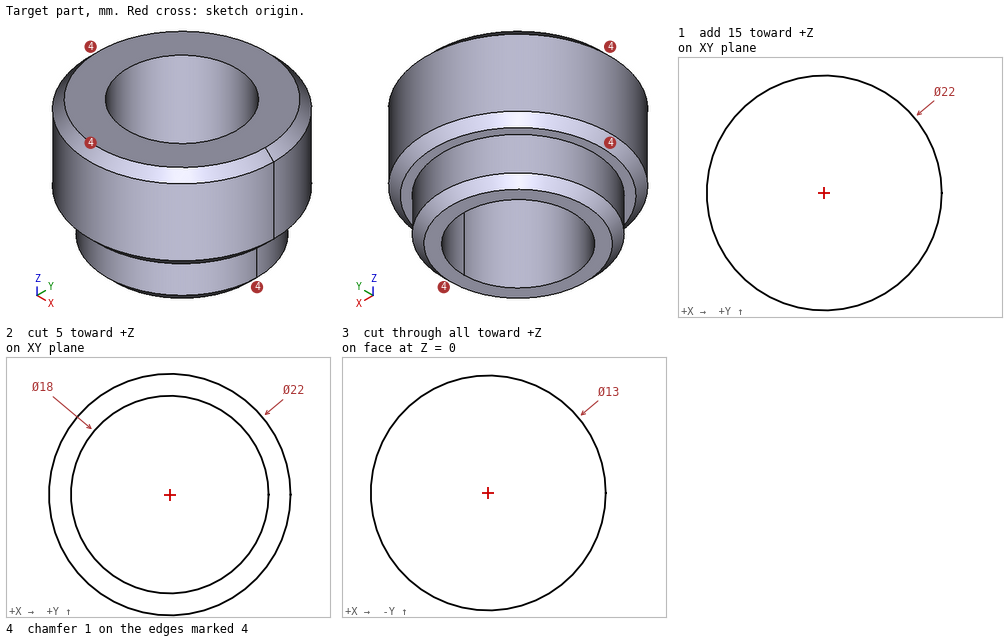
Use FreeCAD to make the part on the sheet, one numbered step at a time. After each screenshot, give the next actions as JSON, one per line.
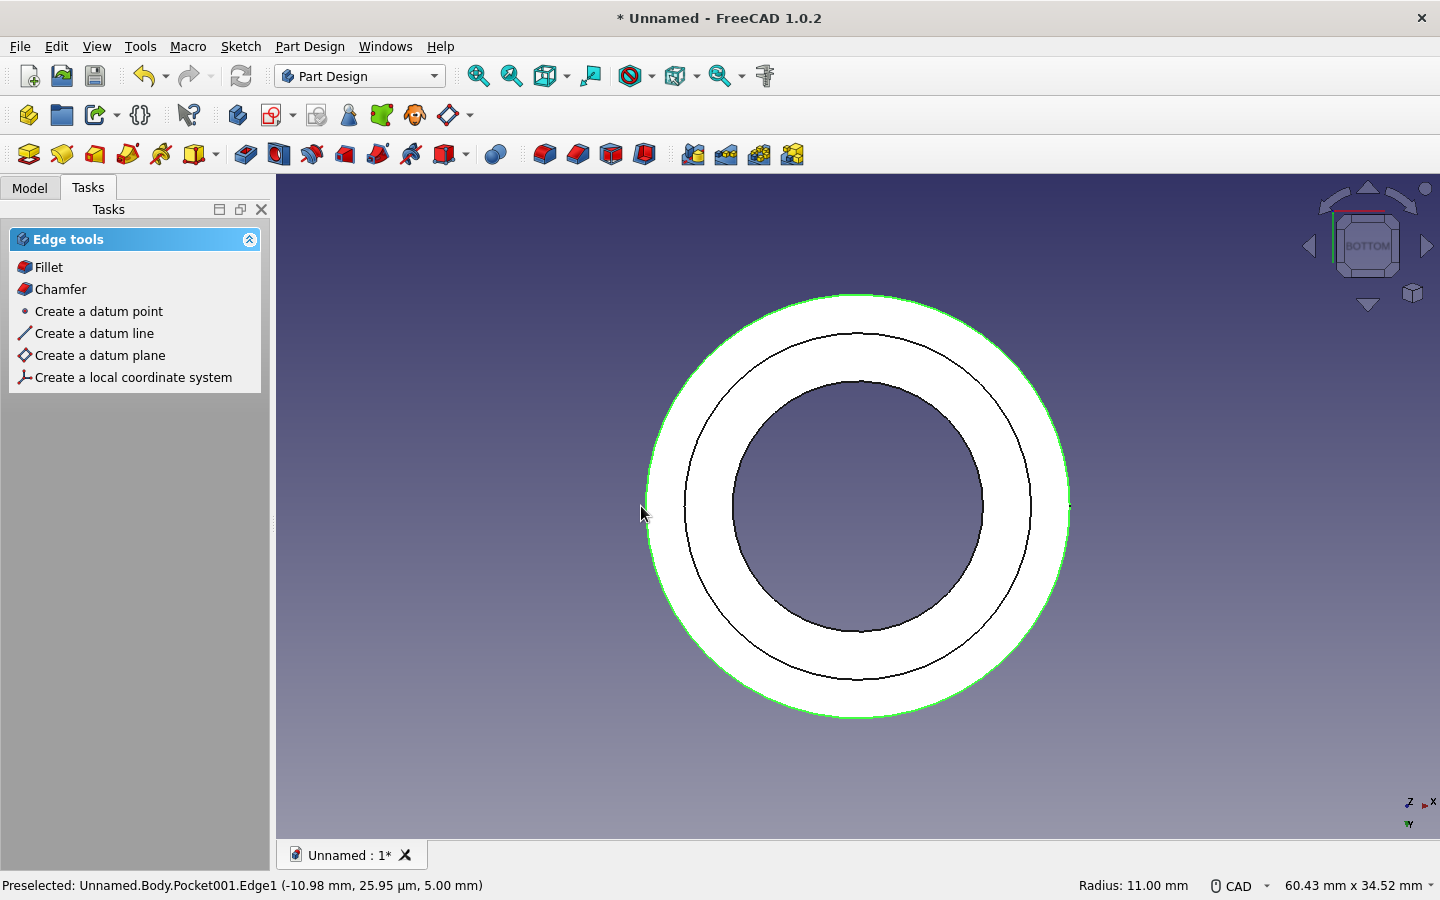
{"action": "left_click", "coordinate": [684, 506], "text": "ctrl"}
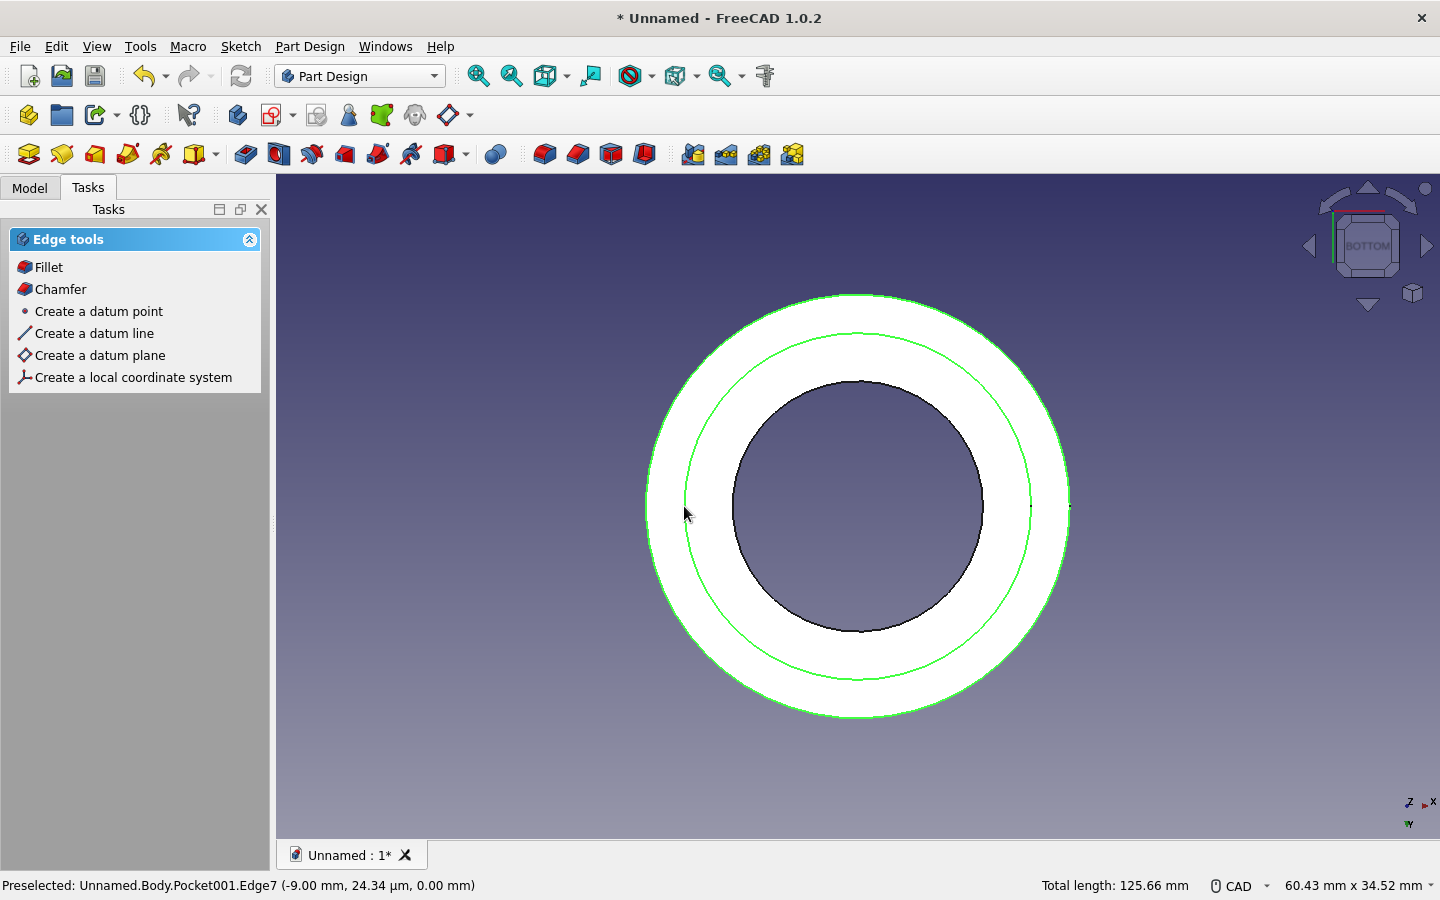
{"action": "key", "text": "0"}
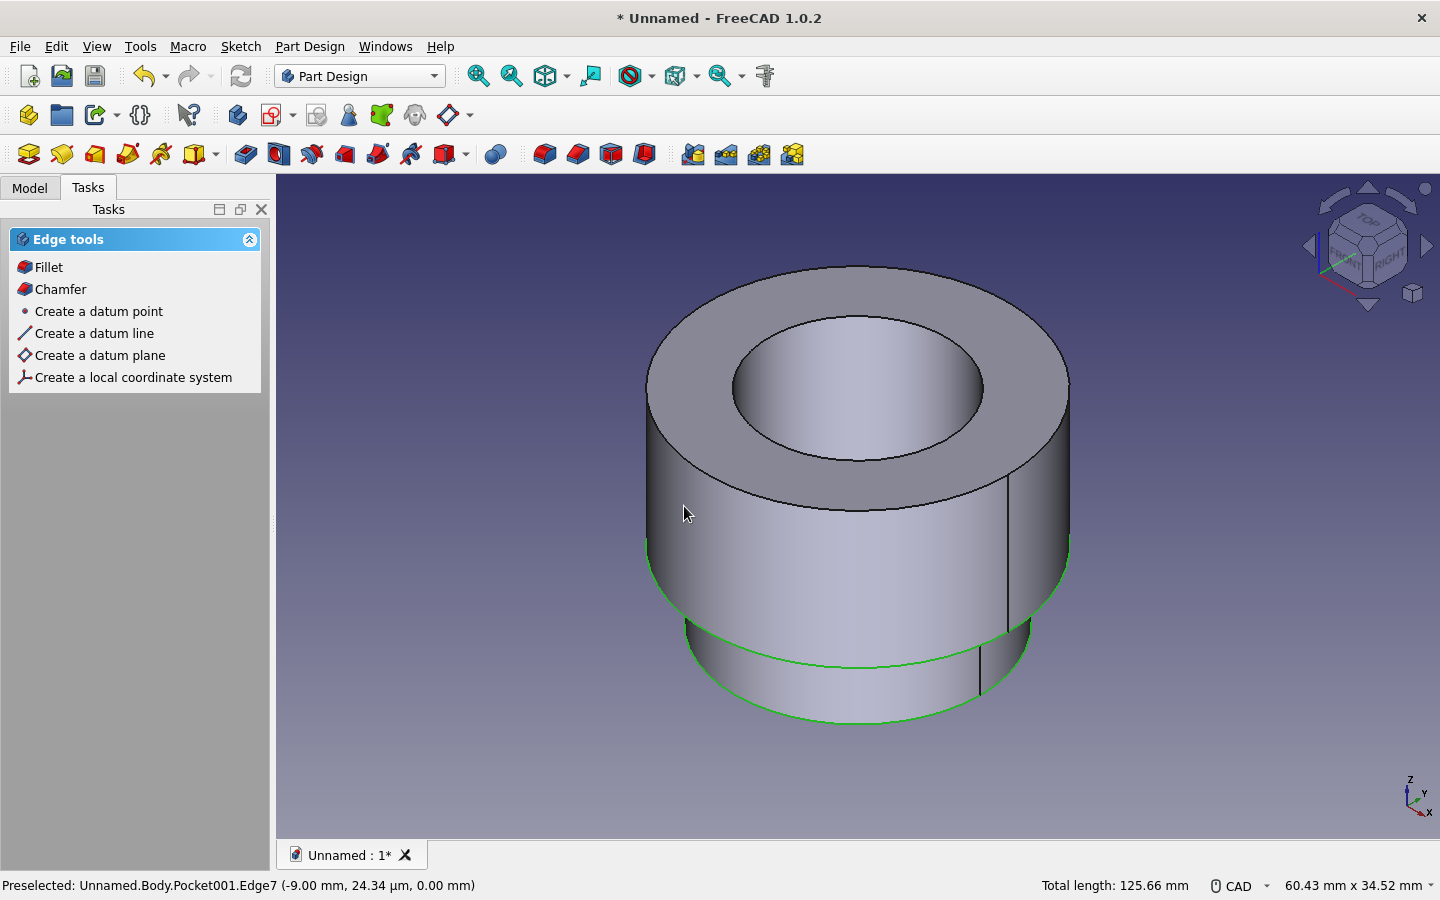
{"action": "left_click", "coordinate": [669, 443], "text": "ctrl"}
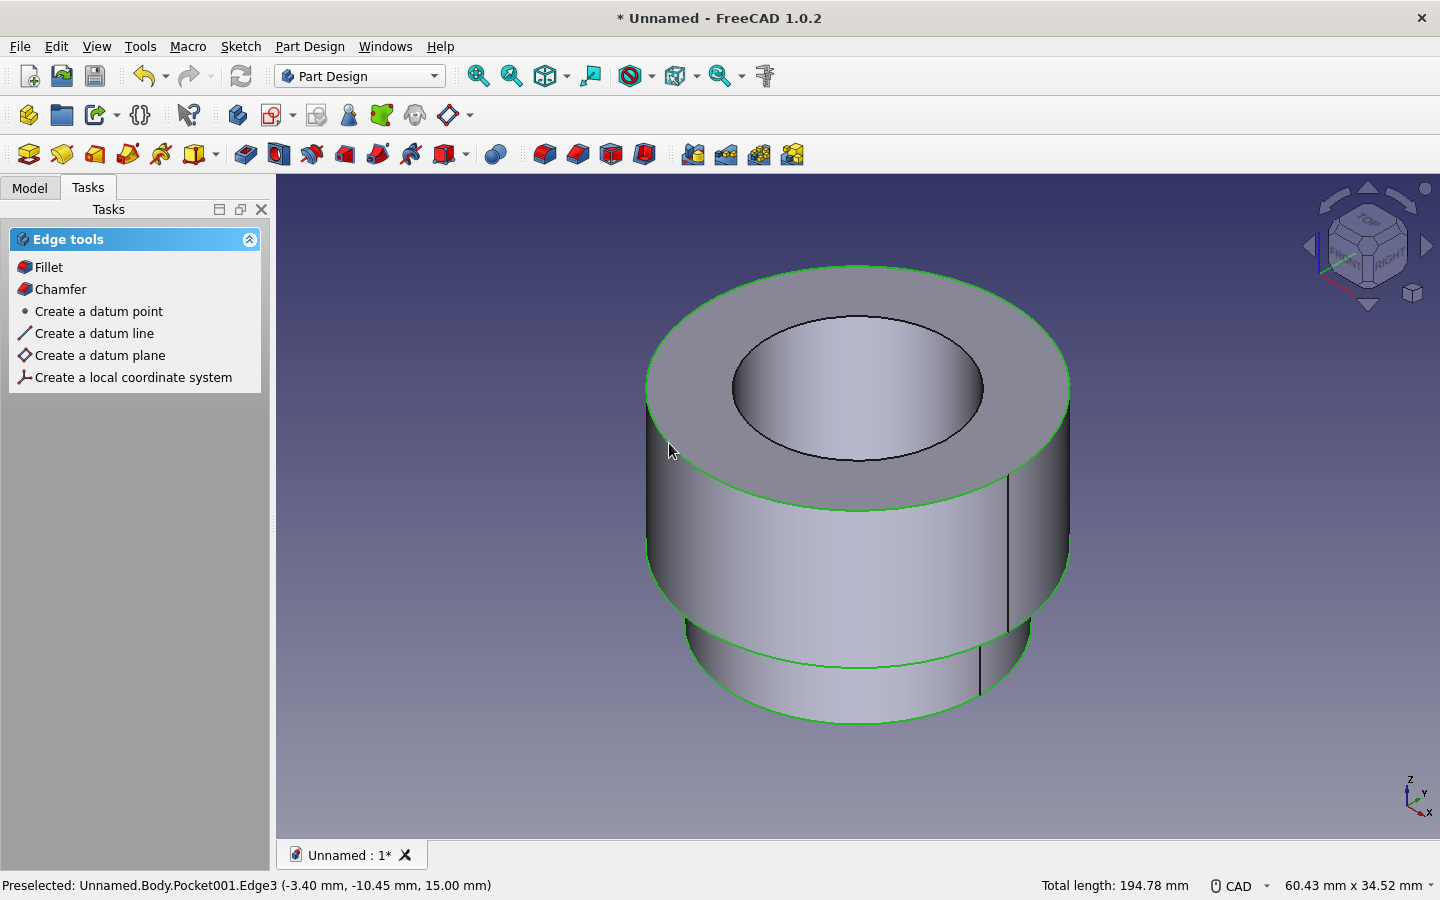
{"action": "left_click", "coordinate": [578, 154]}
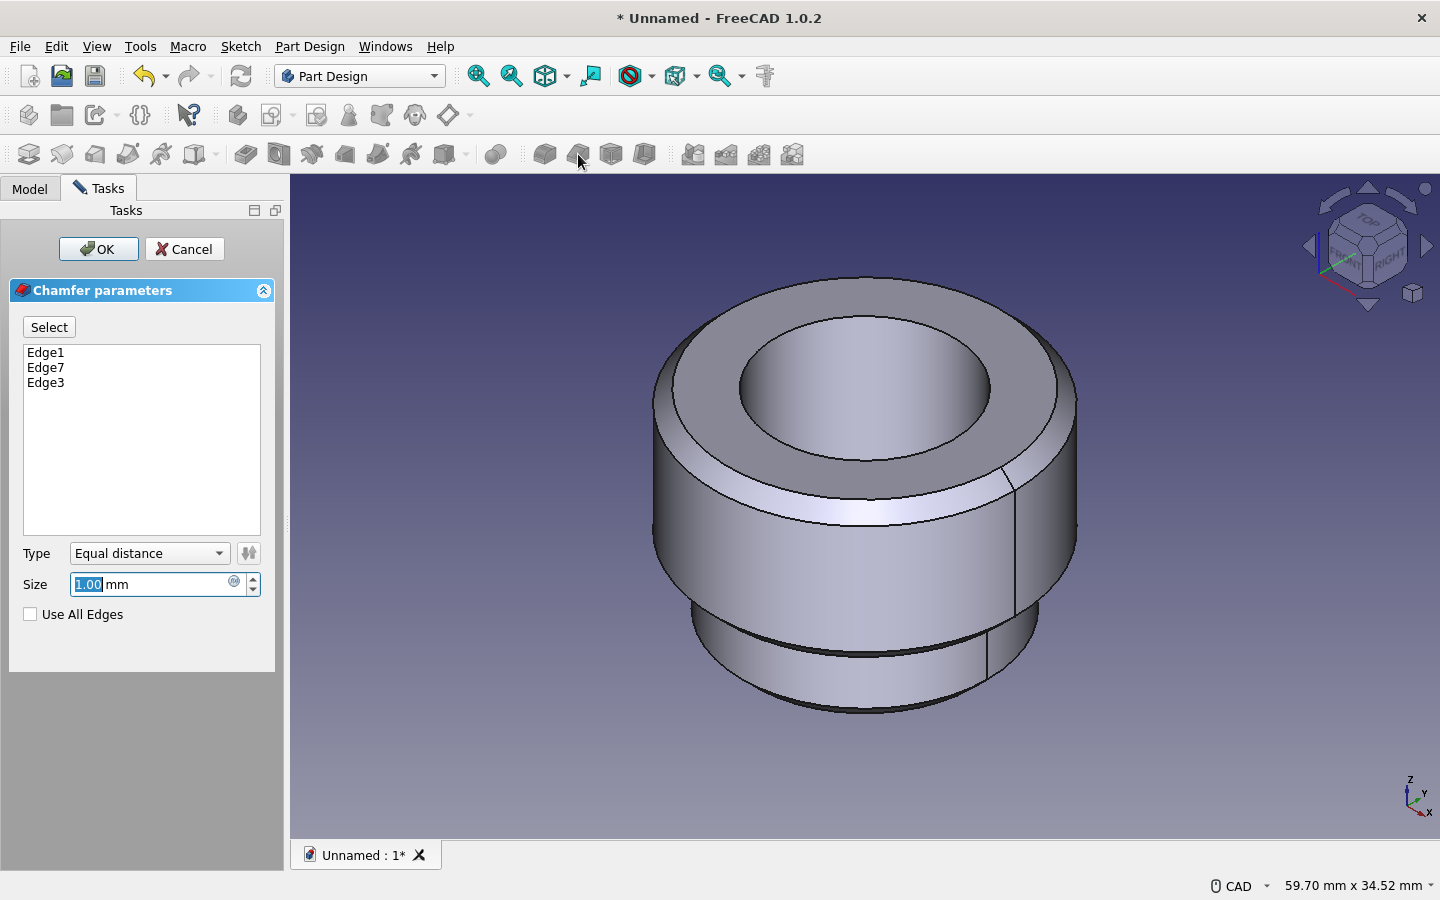
{"action": "type", "text": "1"}
{"action": "key", "text": "Tab"}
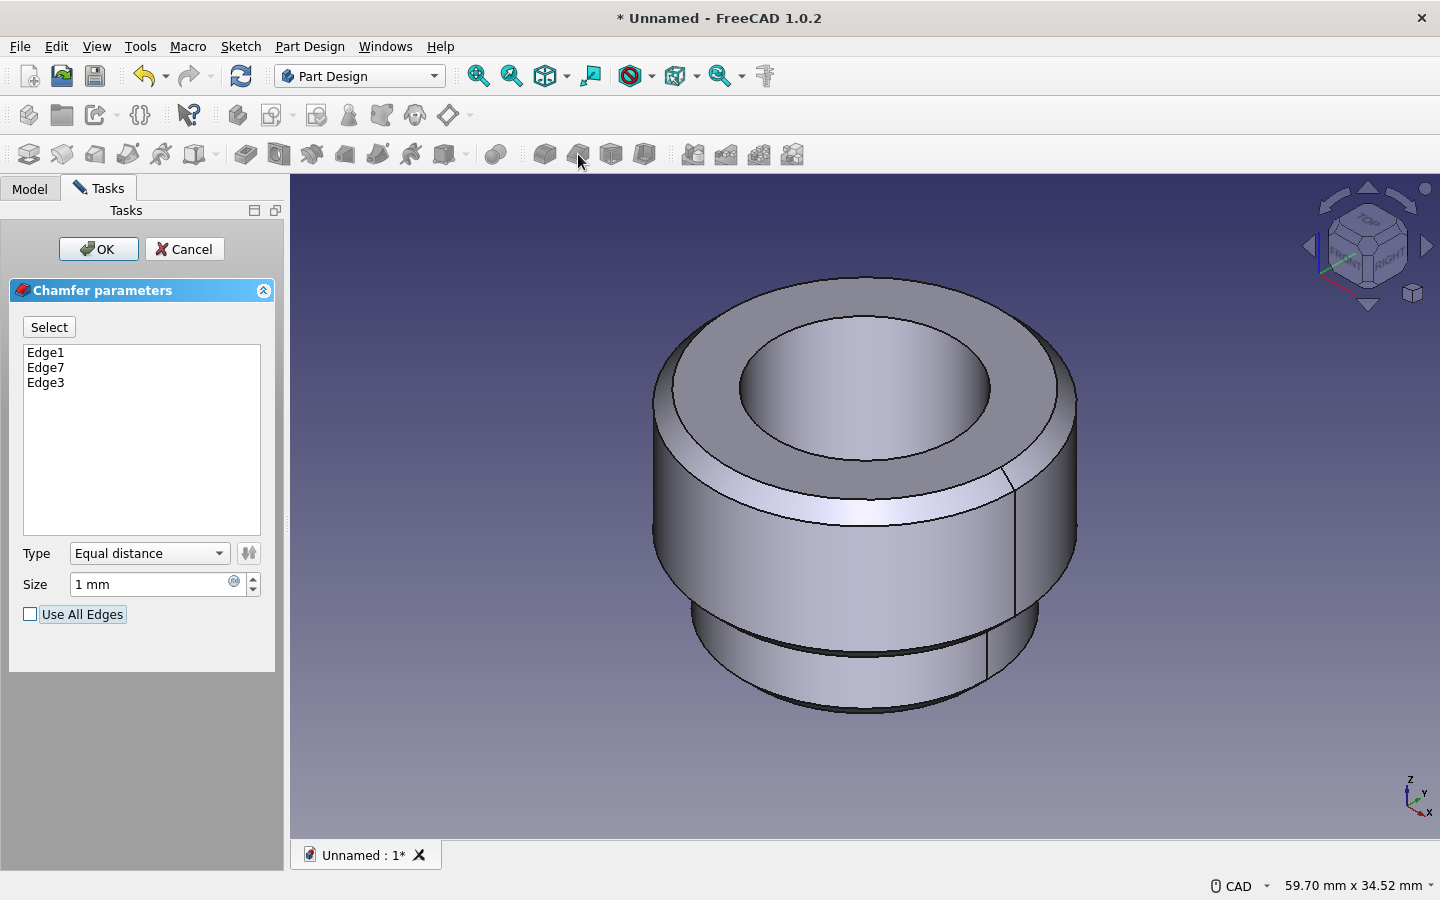
{"action": "left_click", "coordinate": [99, 249]}